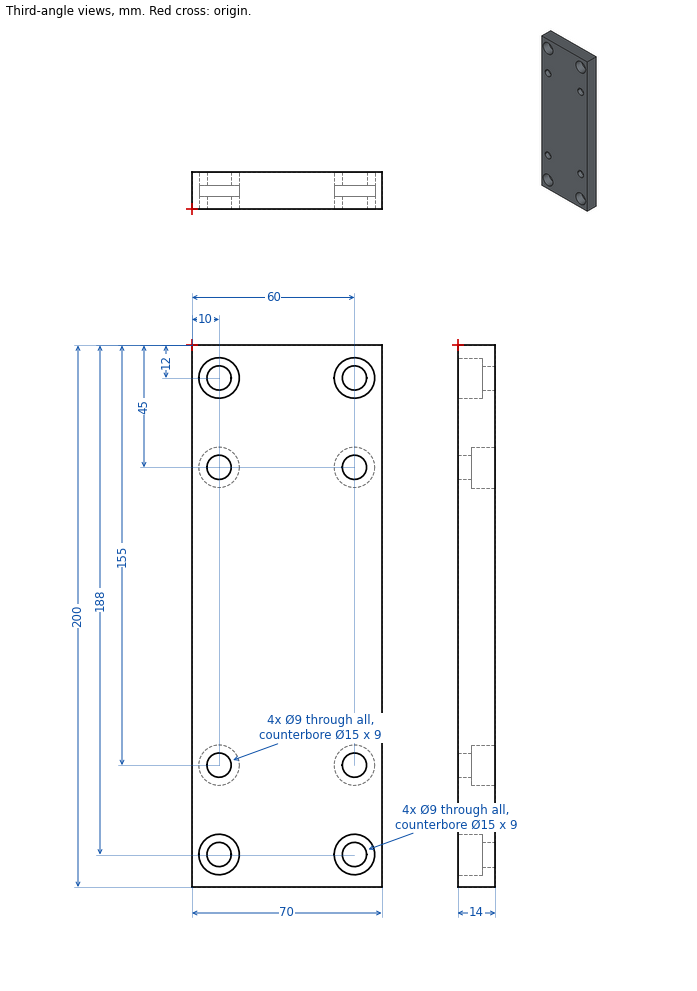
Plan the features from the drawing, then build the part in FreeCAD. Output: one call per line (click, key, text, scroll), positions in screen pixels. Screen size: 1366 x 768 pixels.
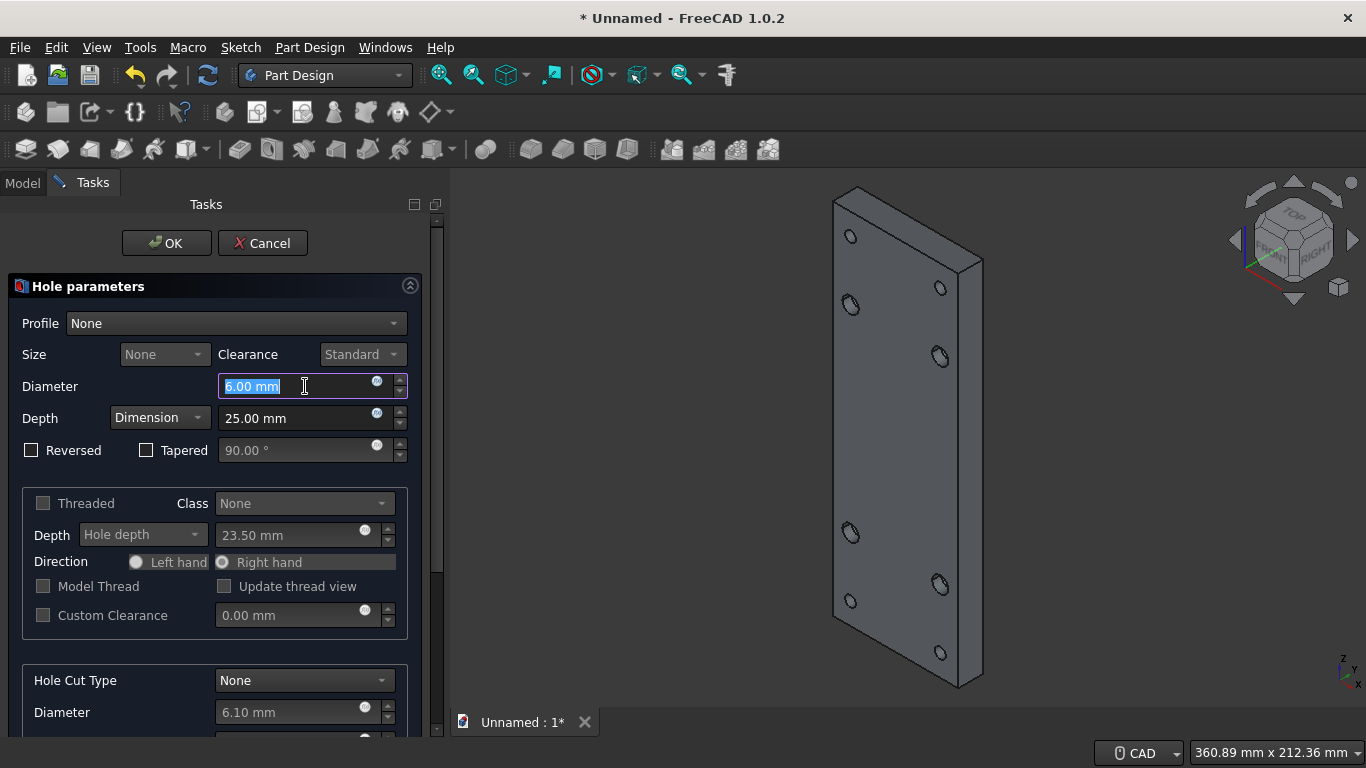
text(9)
key(Tab)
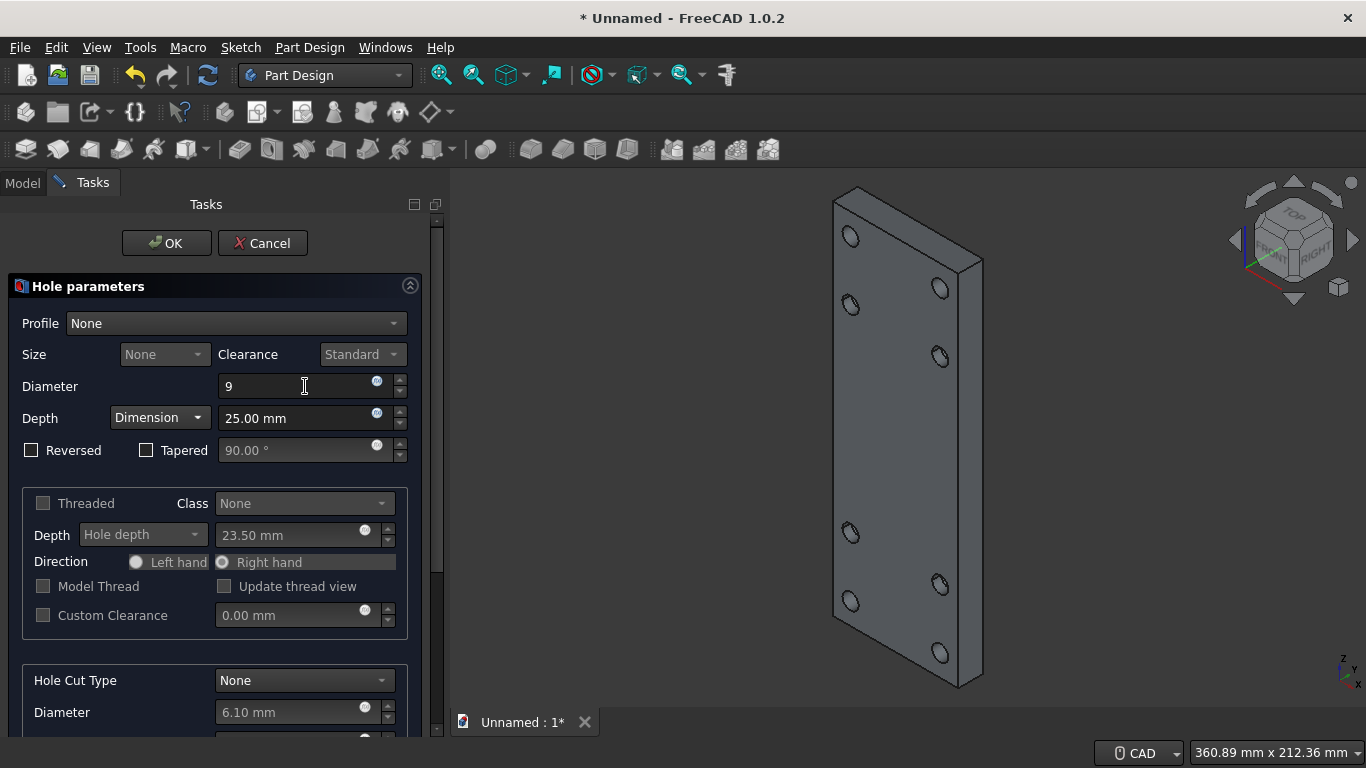
click(161, 418)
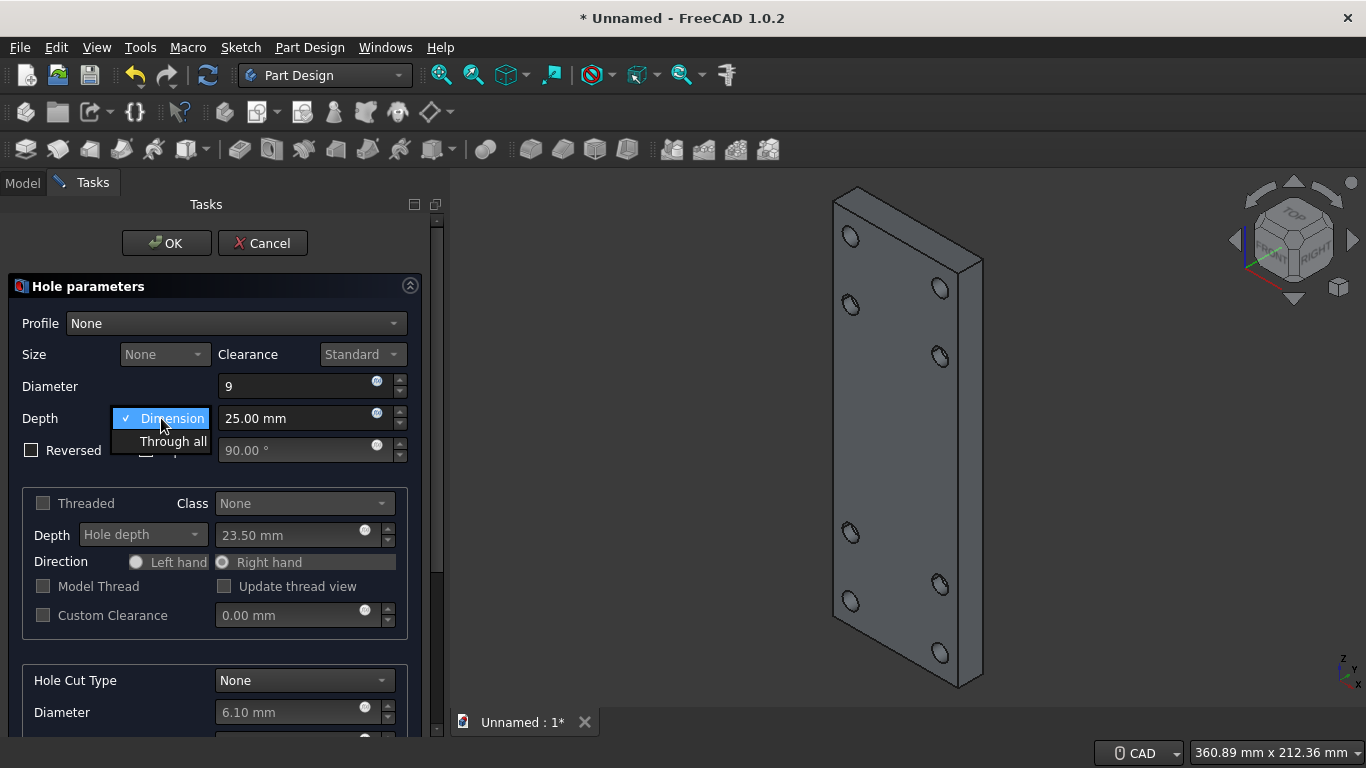
click(160, 442)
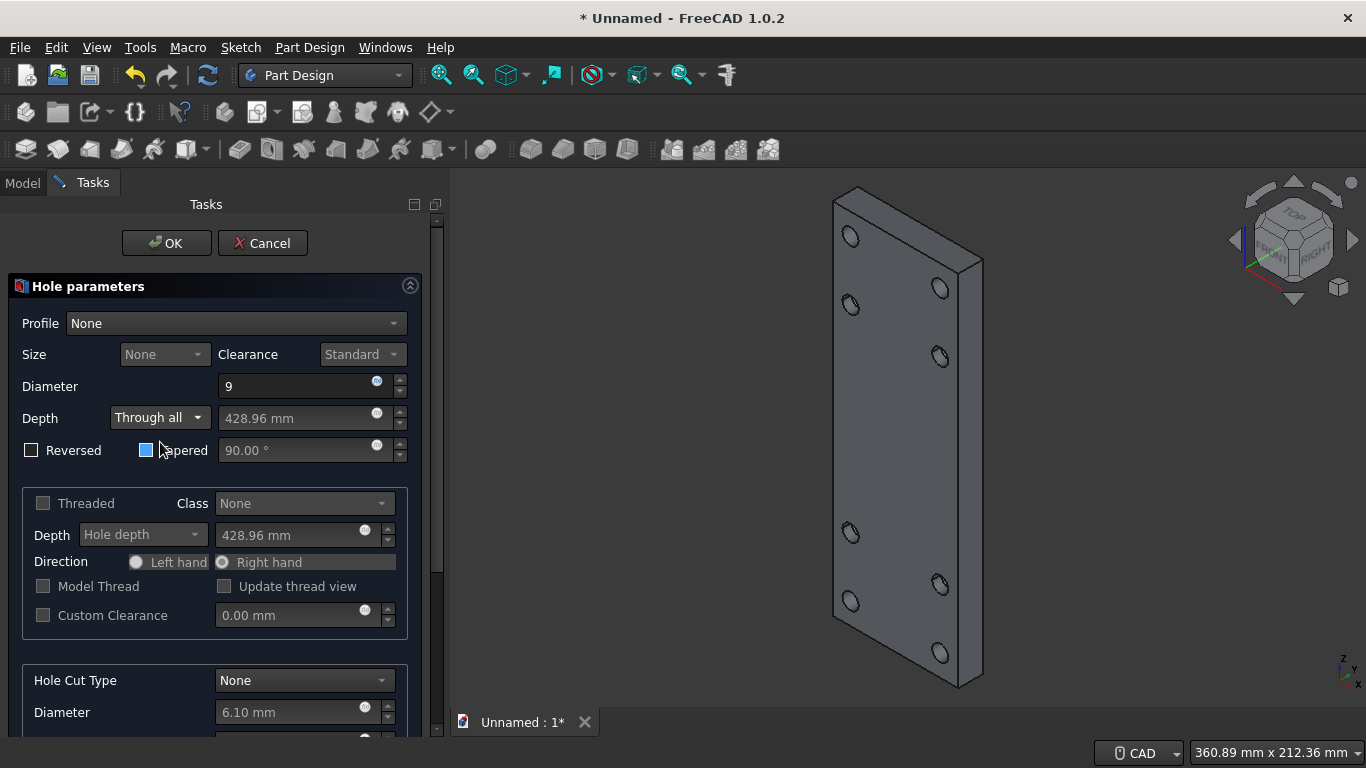
click(306, 680)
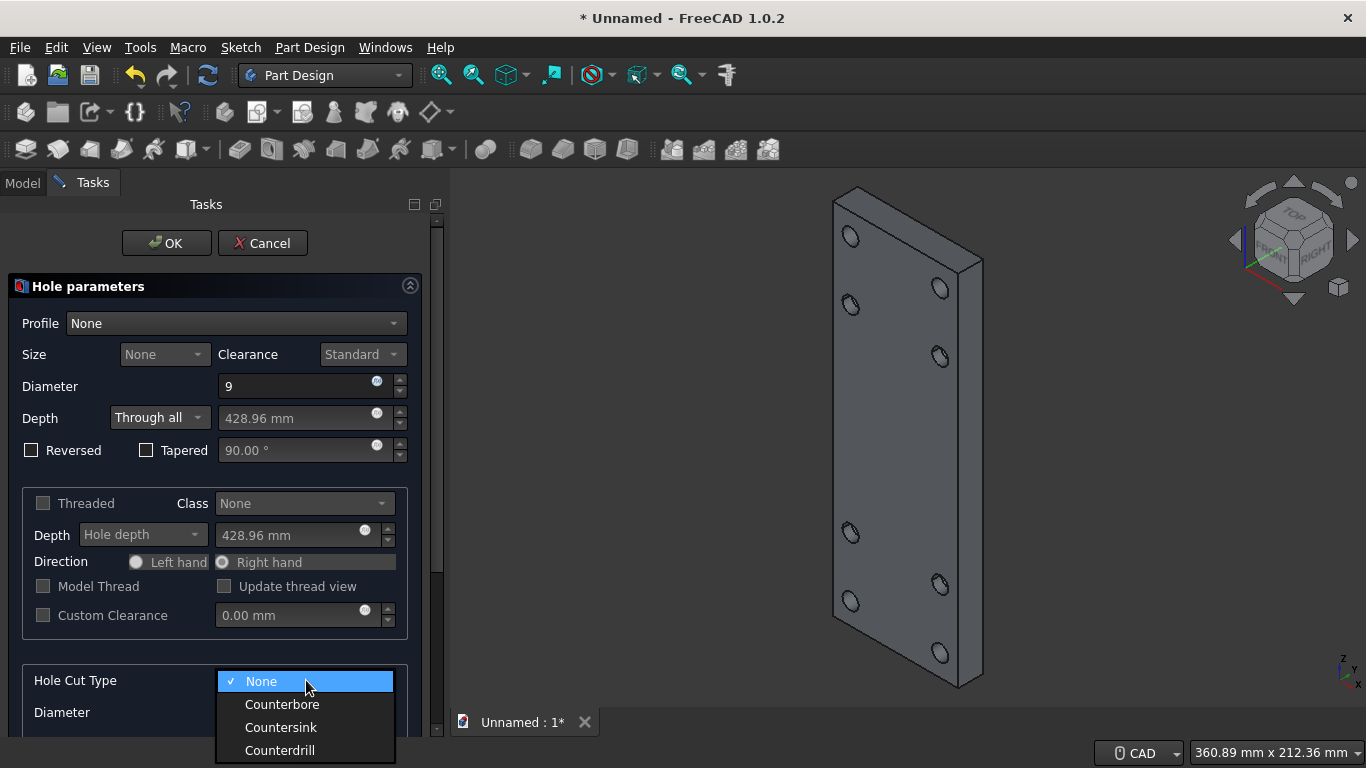
click(304, 704)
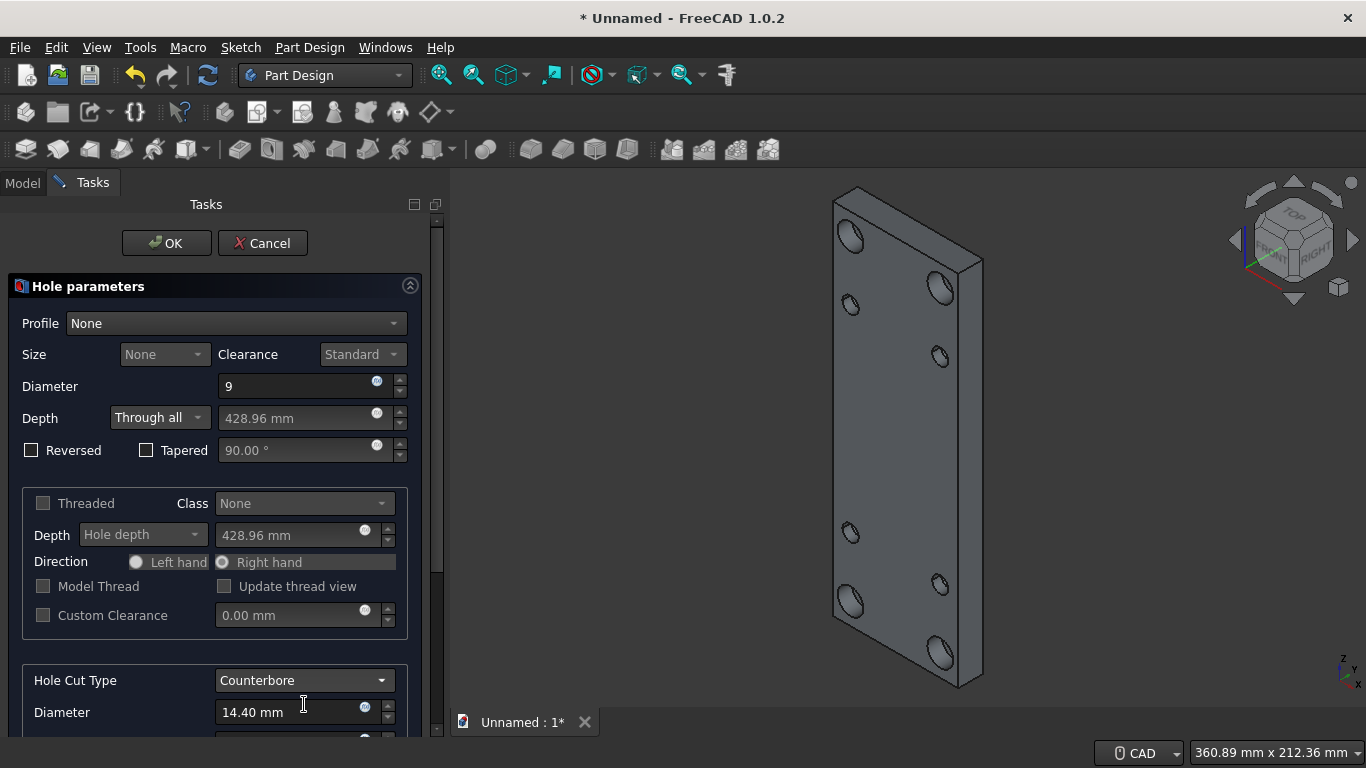
triple_click(298, 712)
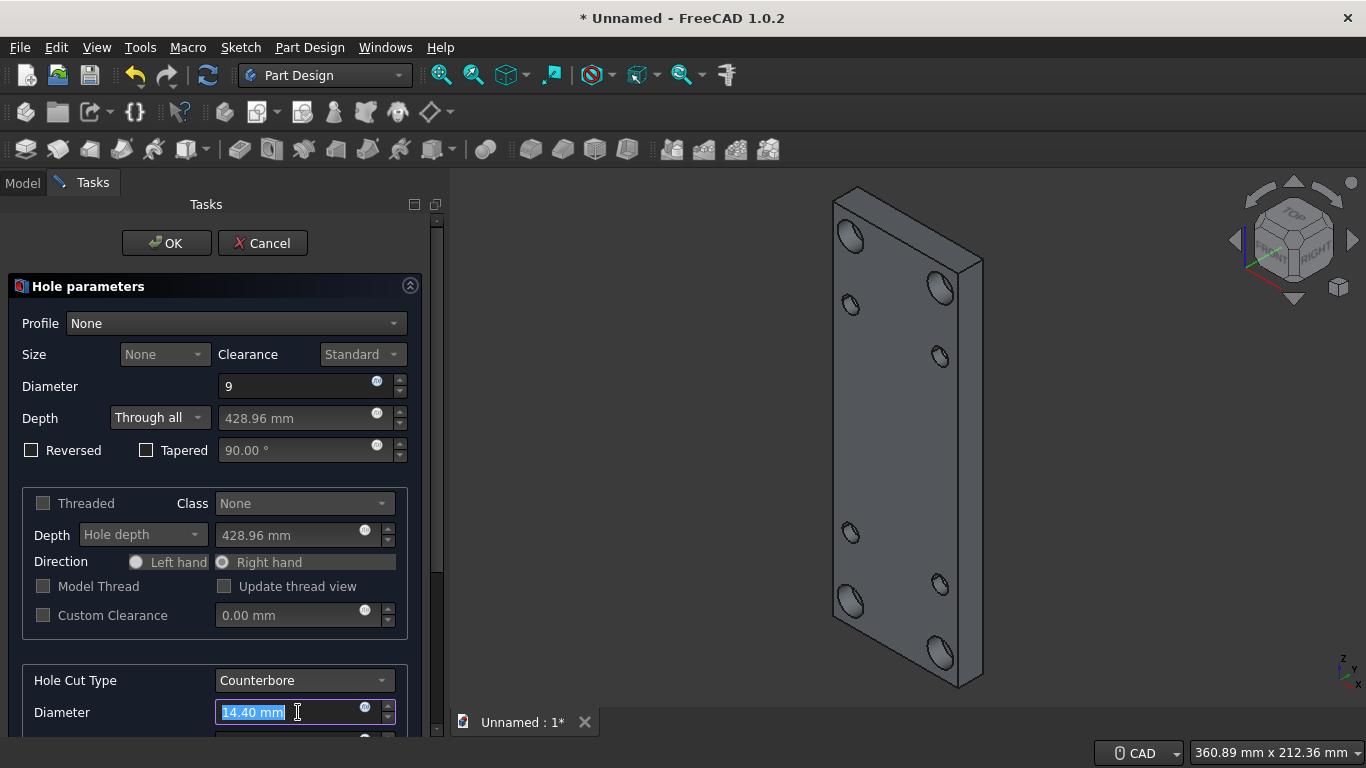
text(15)
key(Tab)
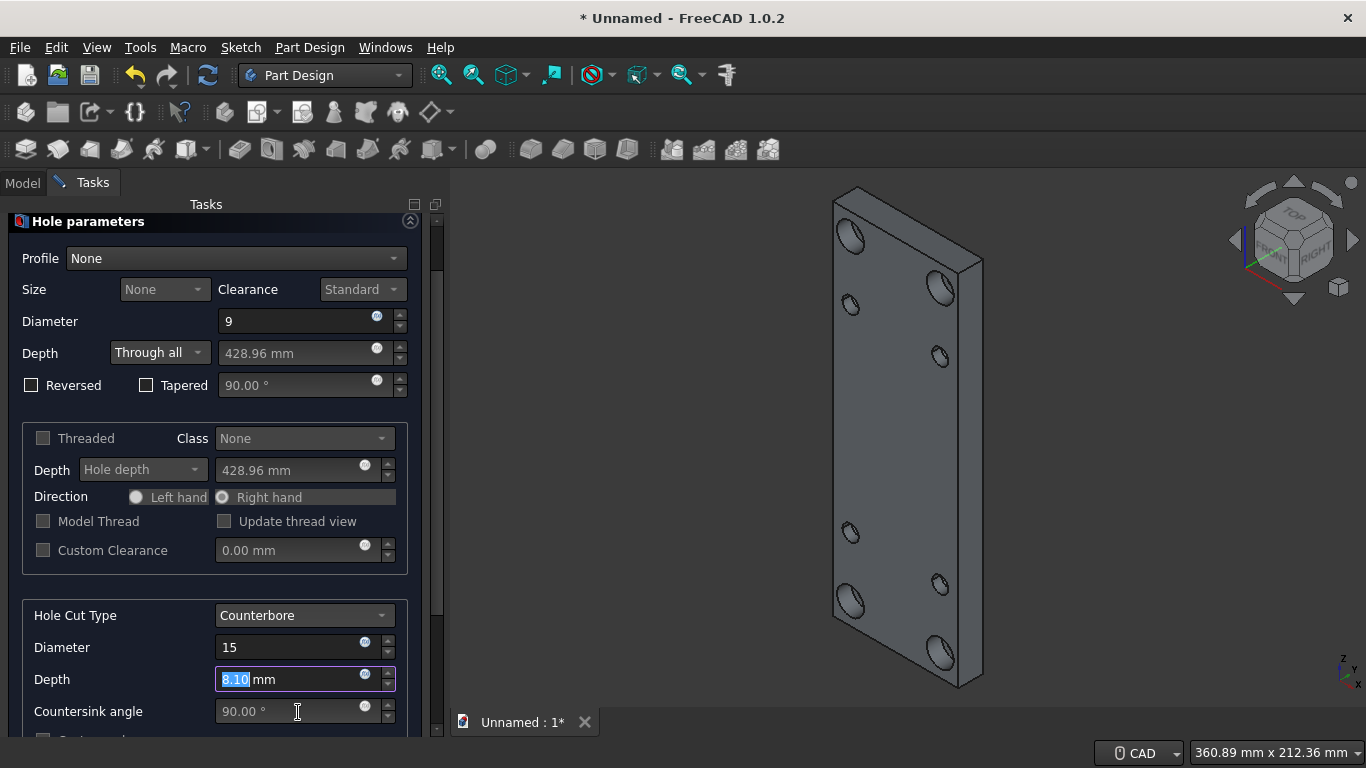
text(9)
key(Tab)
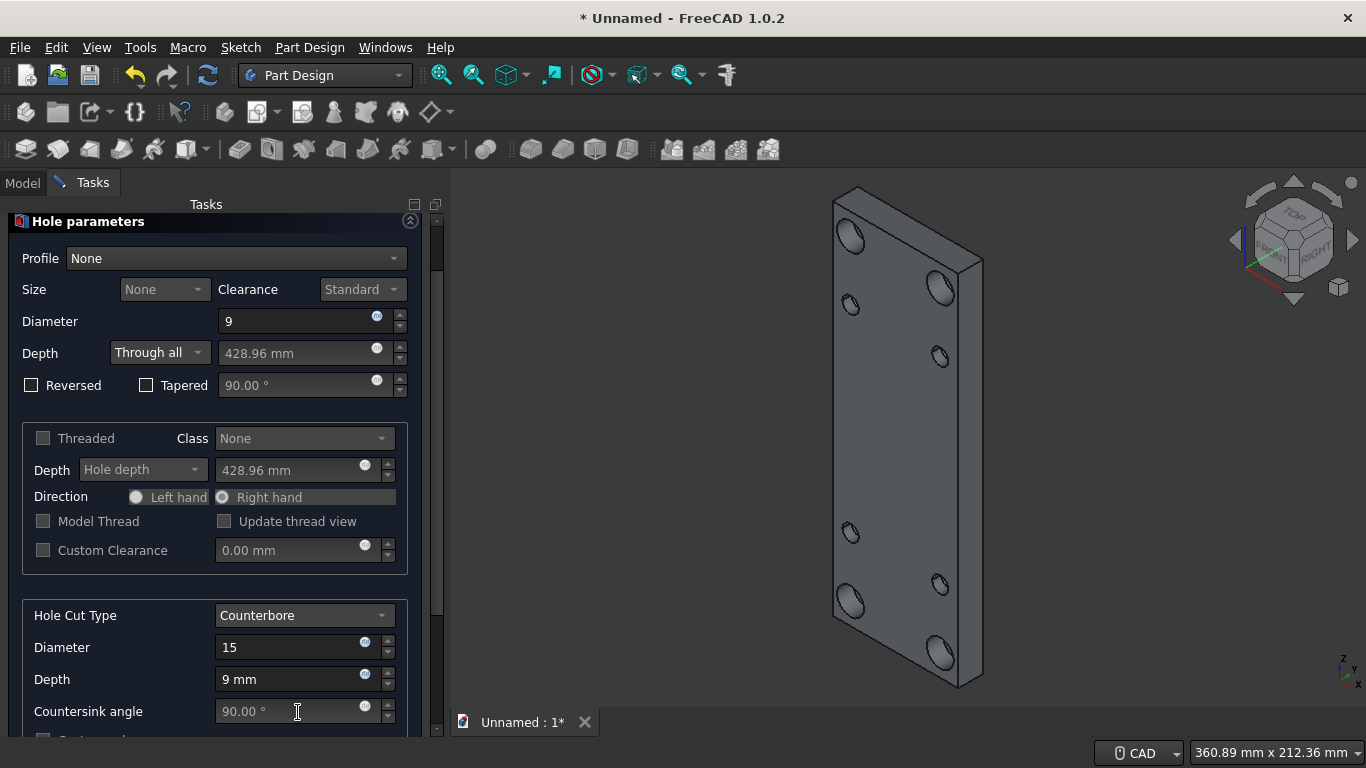
scroll(437, 475, up, 2)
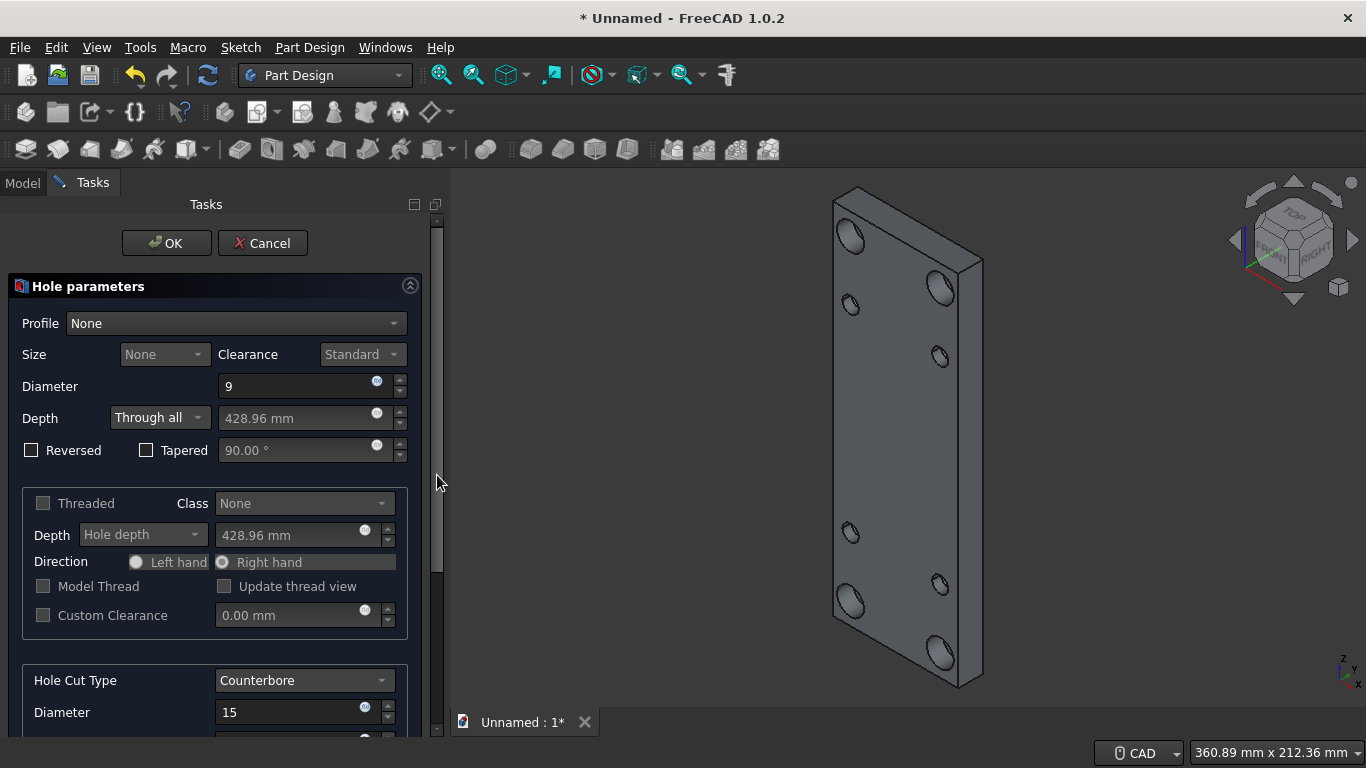
click(167, 243)